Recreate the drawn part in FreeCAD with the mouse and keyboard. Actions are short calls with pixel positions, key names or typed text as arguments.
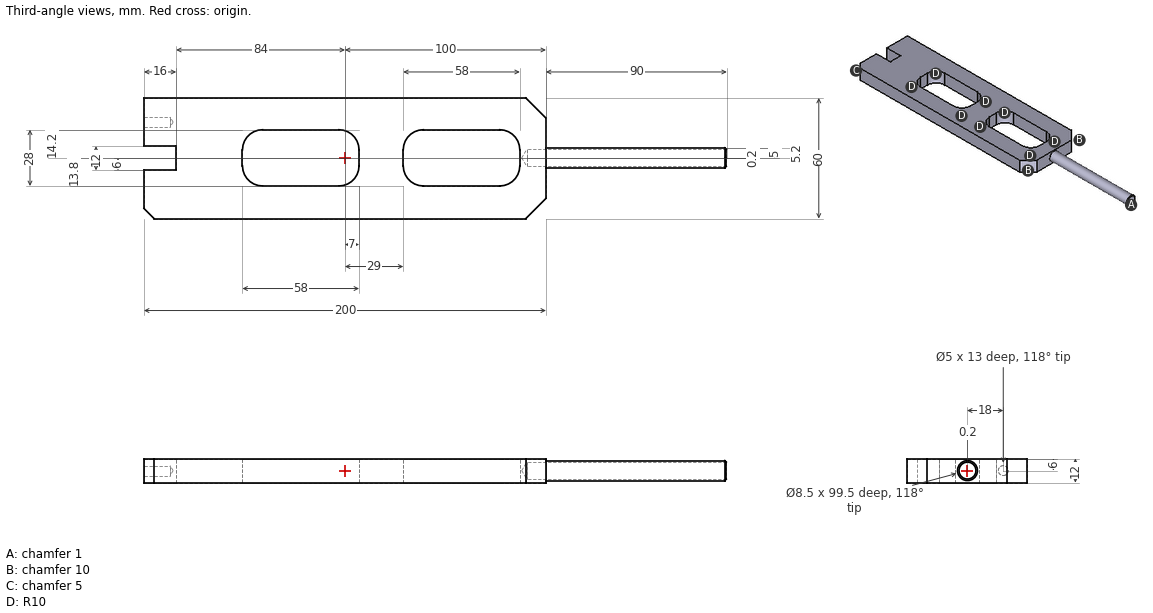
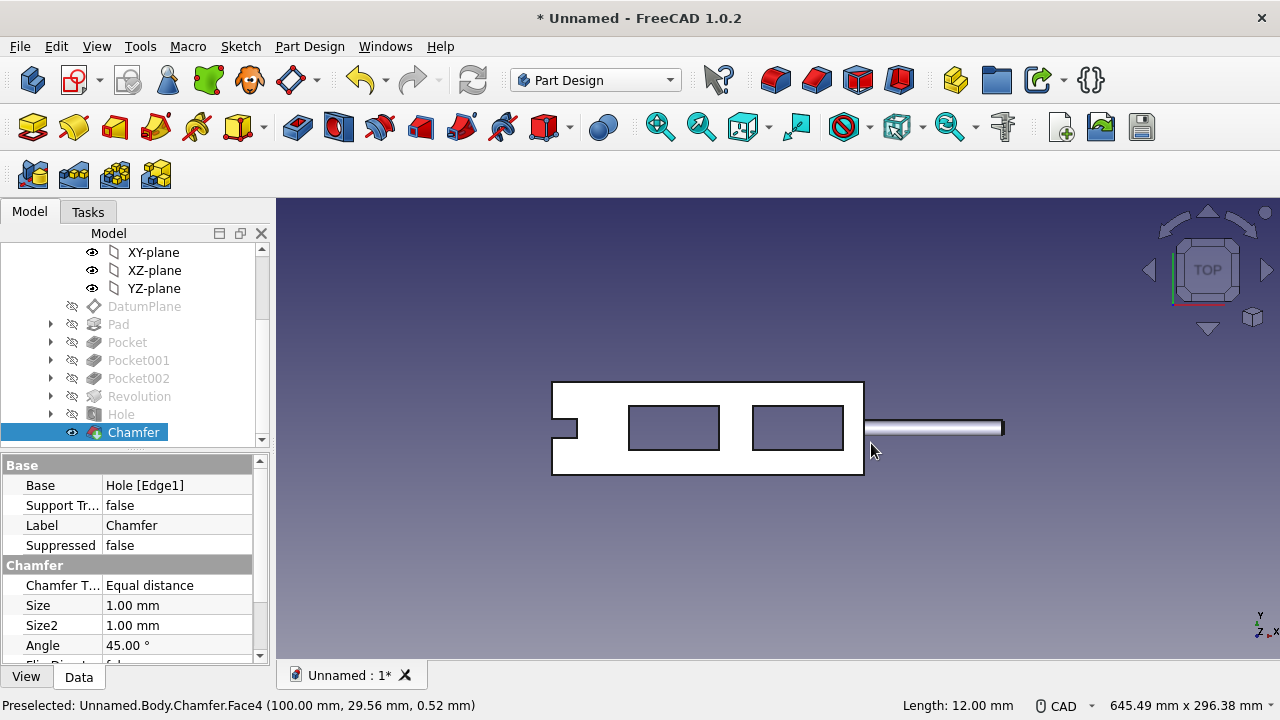
scroll(864, 381, up, 4)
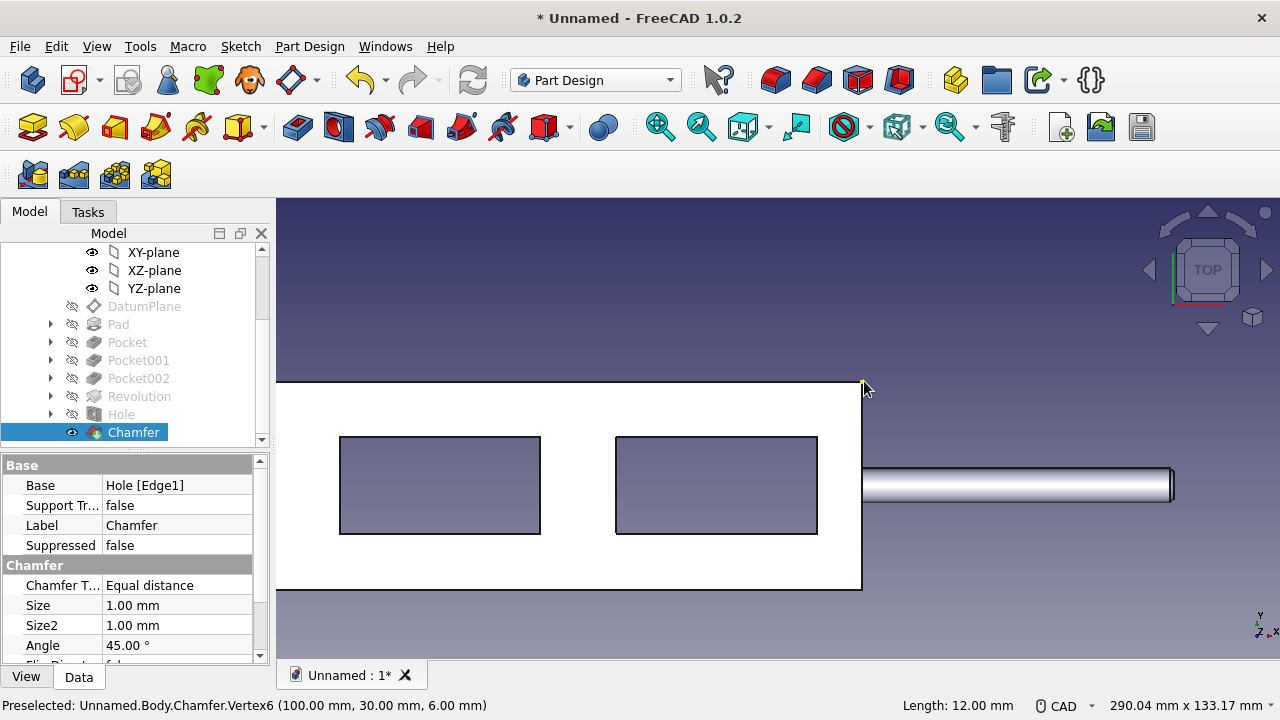
key(v)
key(f)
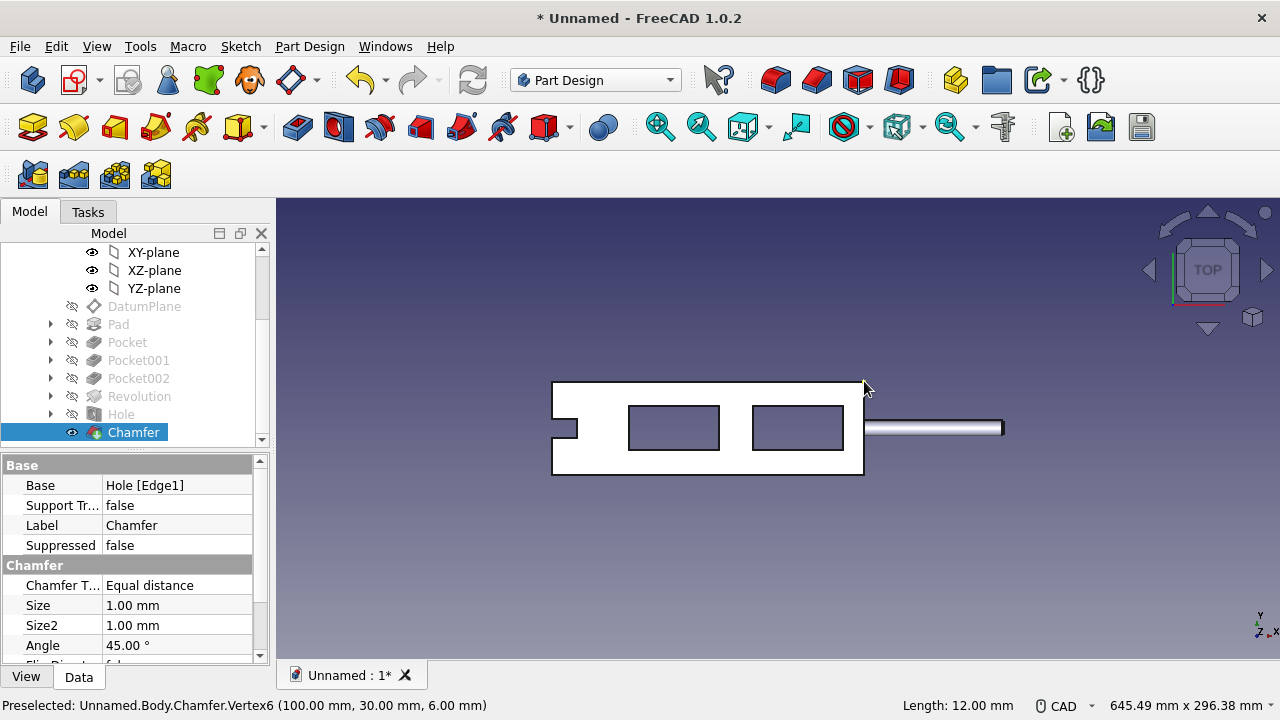
key(0)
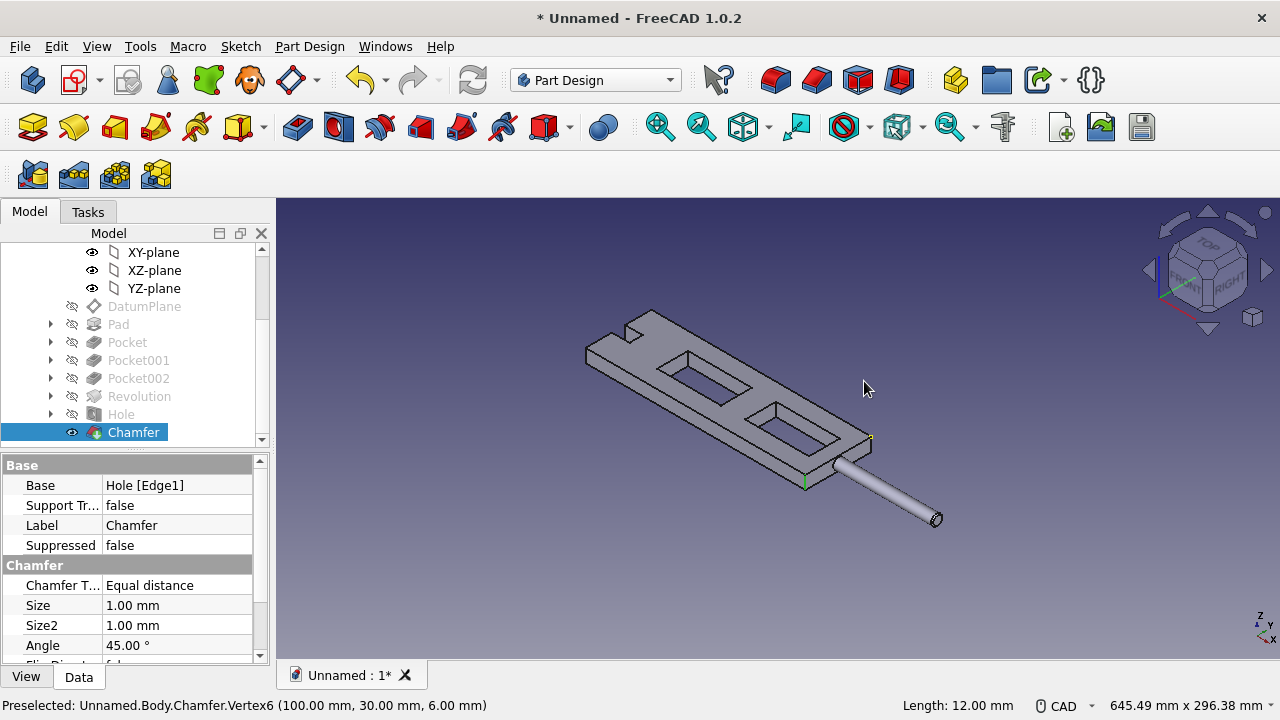
scroll(871, 443, up, 4)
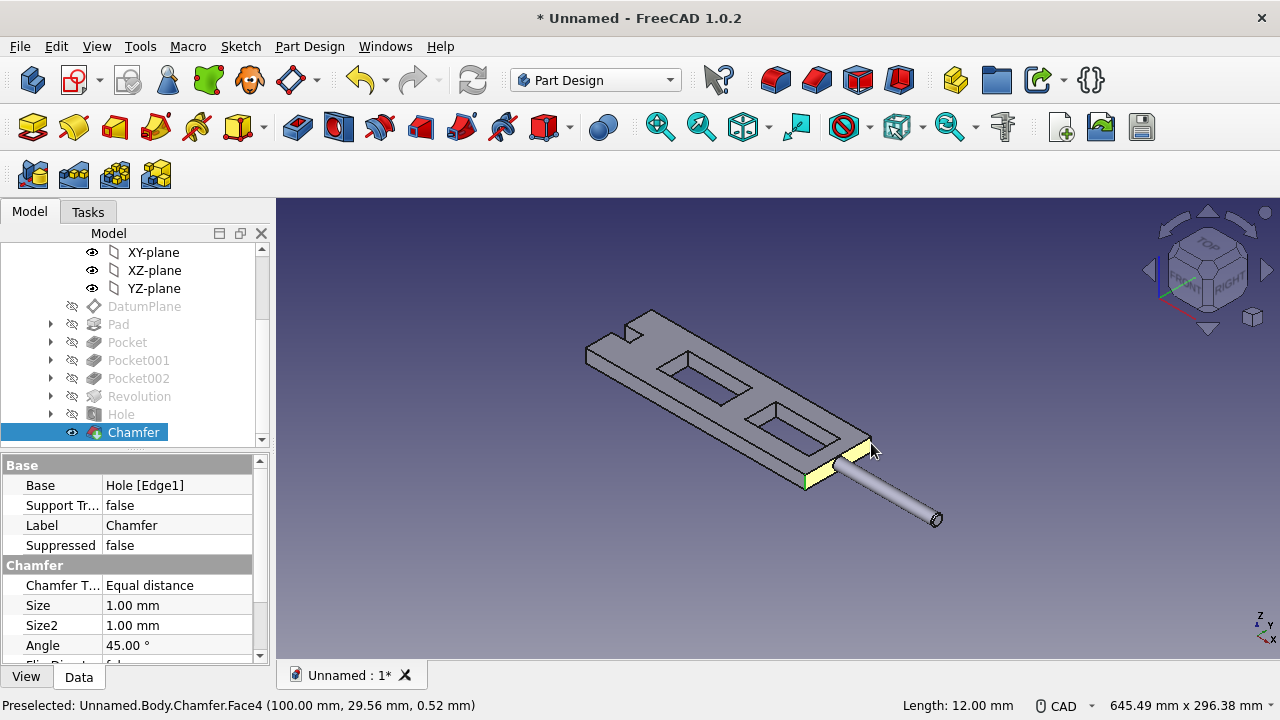
key(v)
key(f)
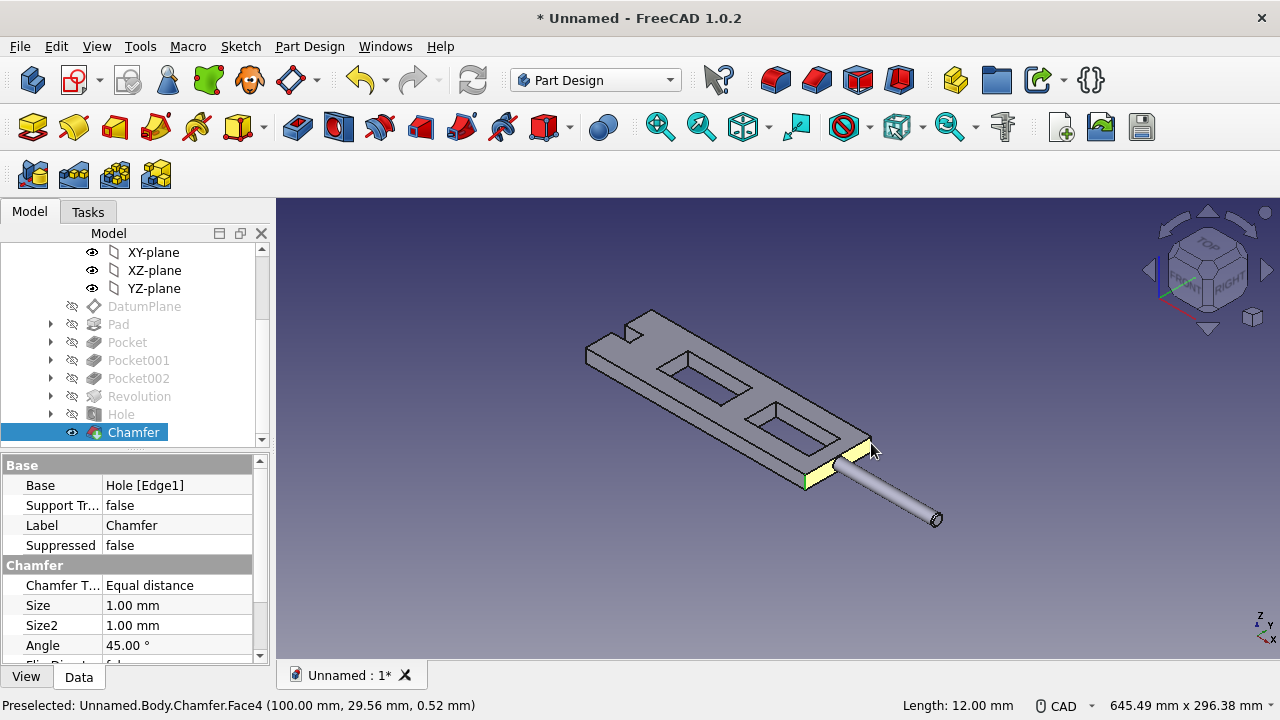
key(1)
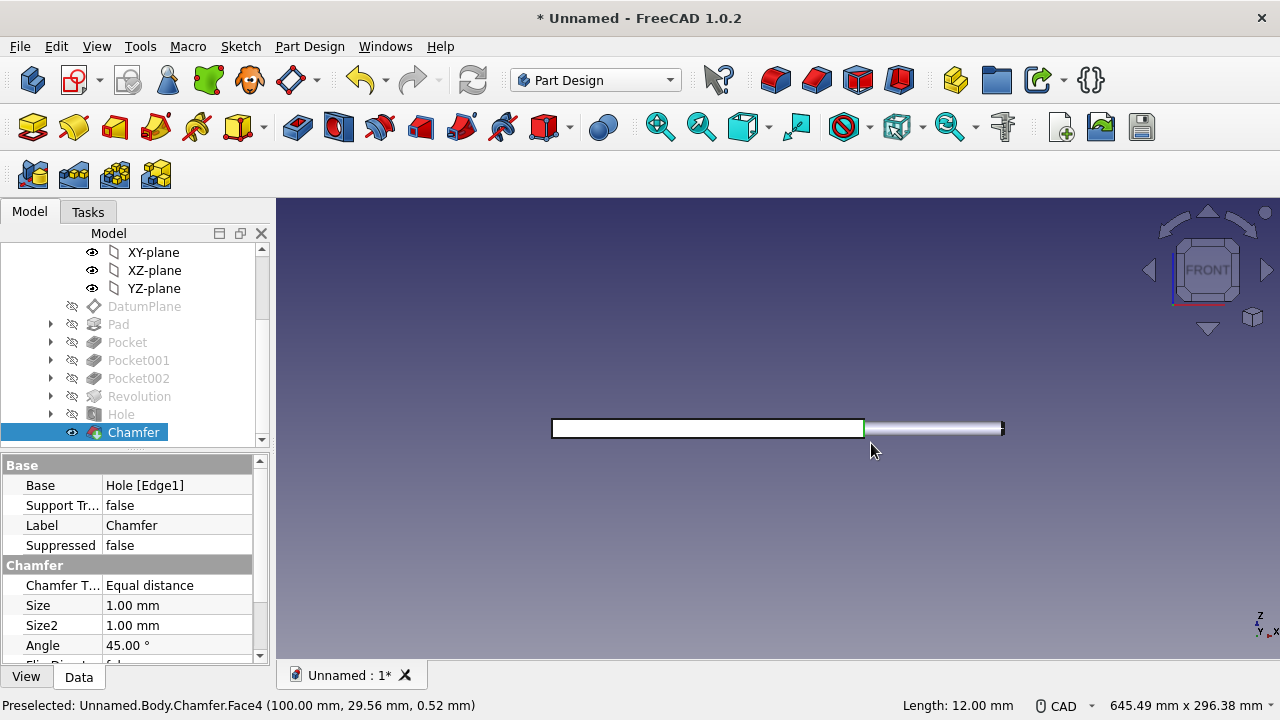
scroll(864, 427, up, 4)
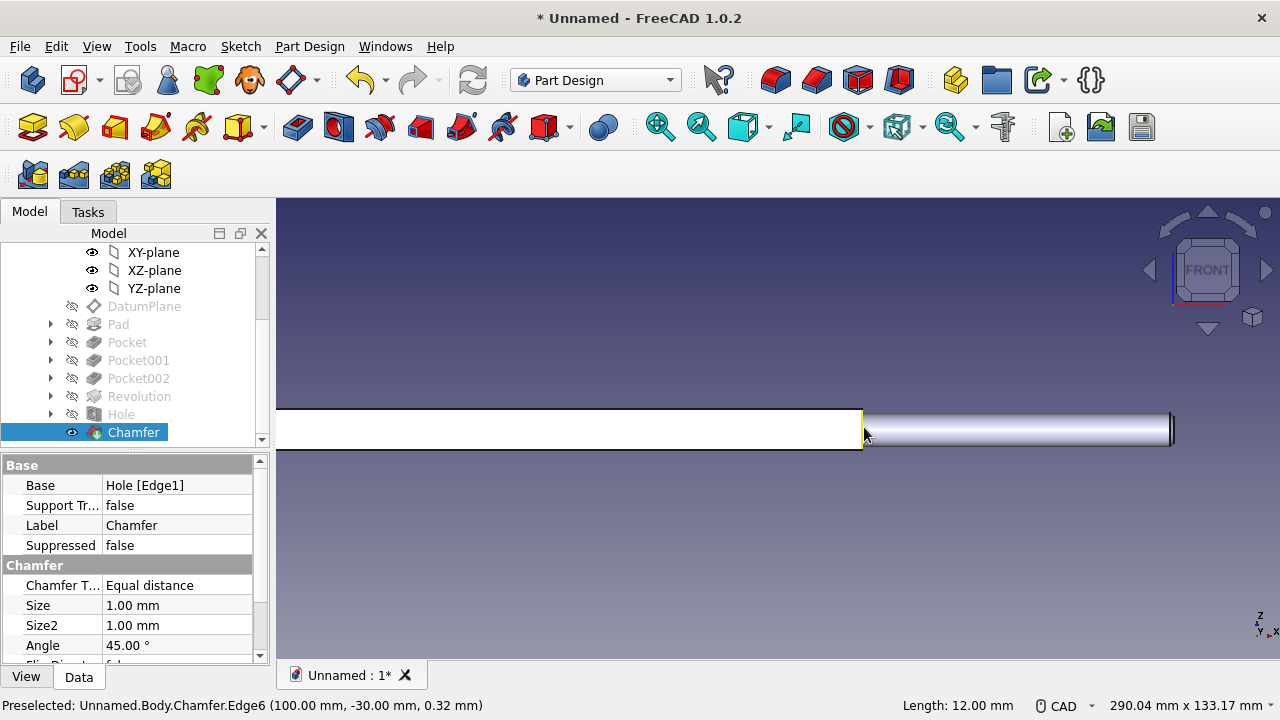
click(661, 128)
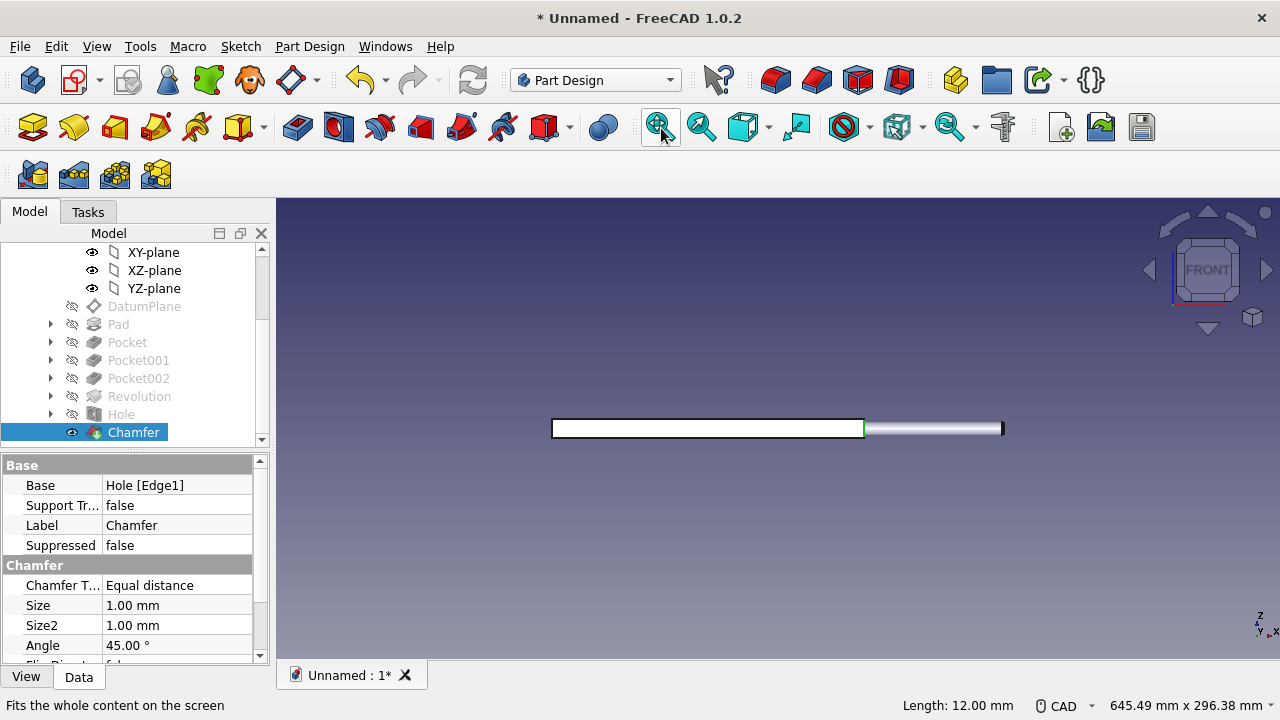
key(3)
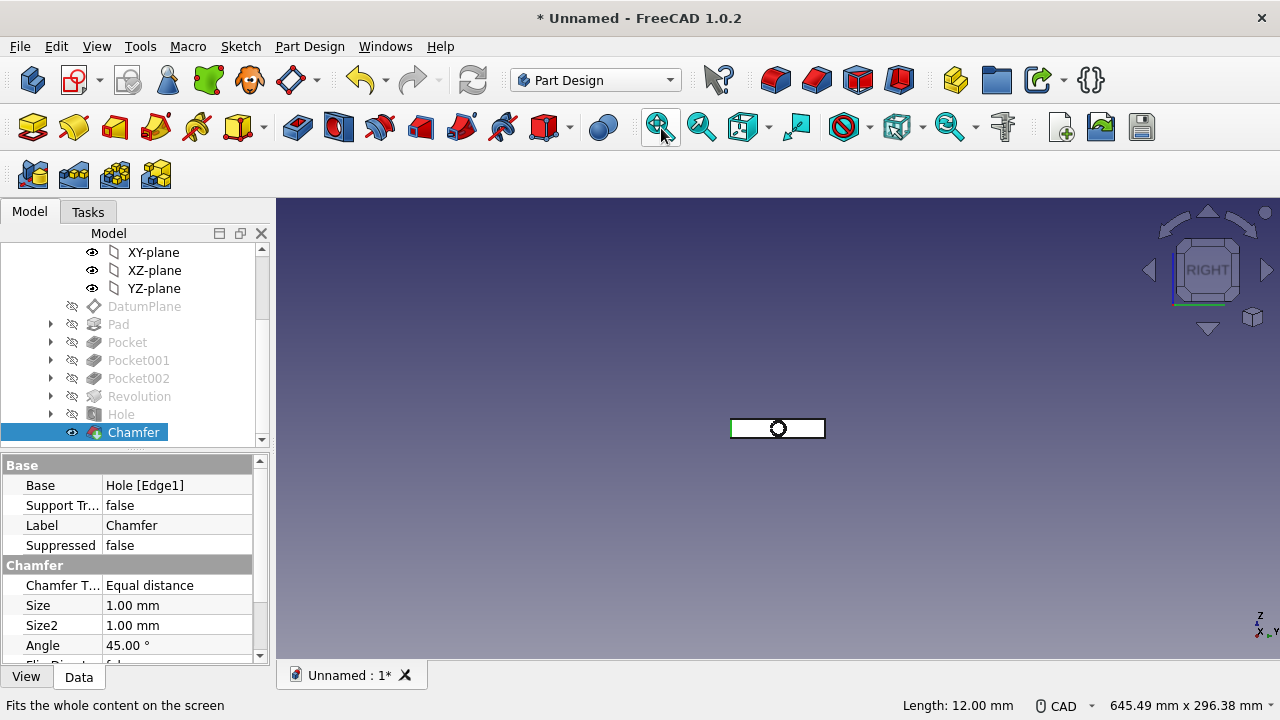
key(v)
key(f)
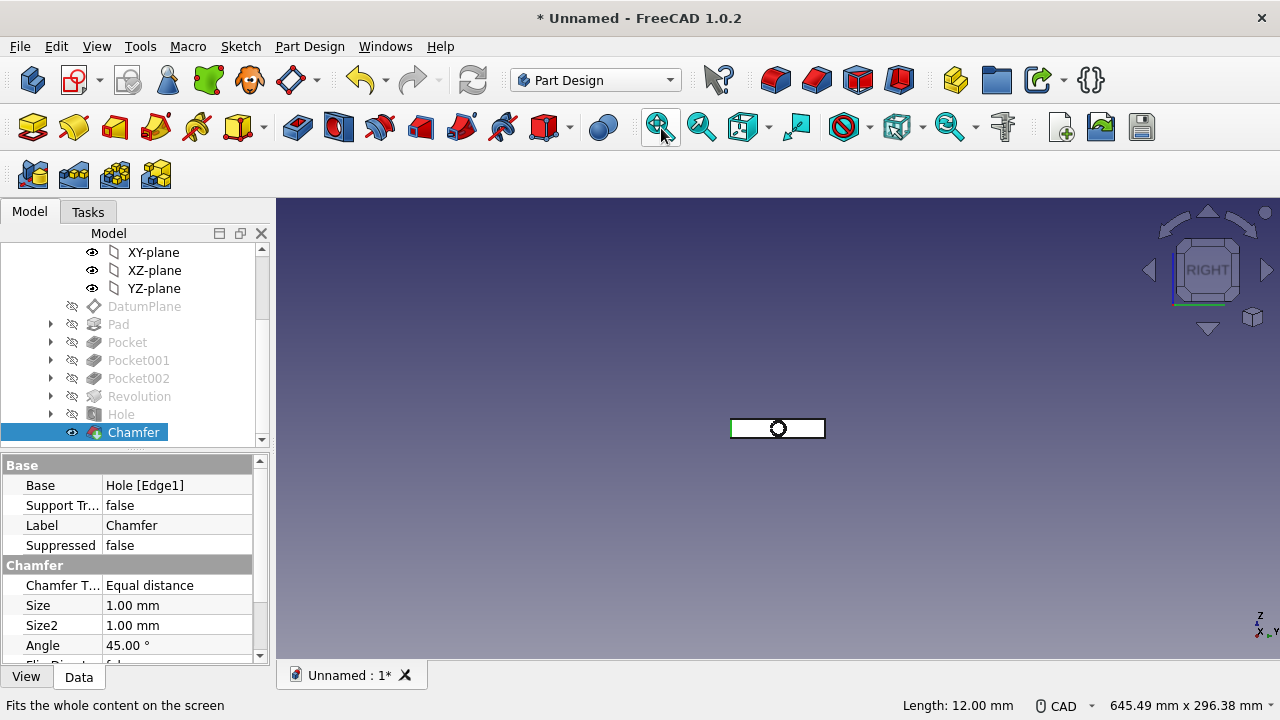
click(825, 427, ctrl)